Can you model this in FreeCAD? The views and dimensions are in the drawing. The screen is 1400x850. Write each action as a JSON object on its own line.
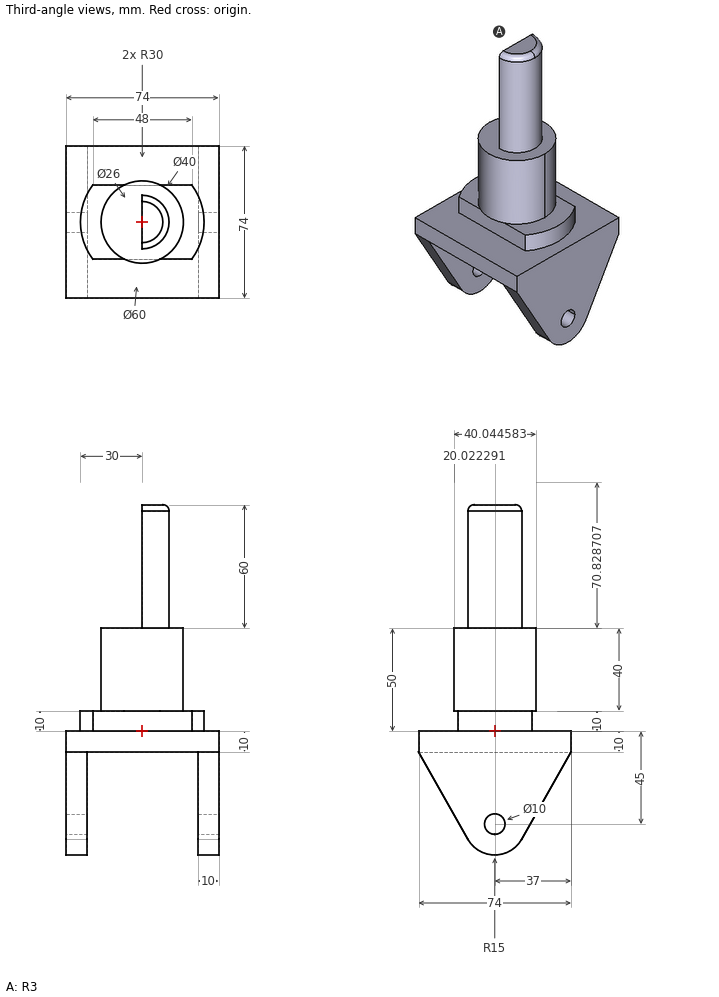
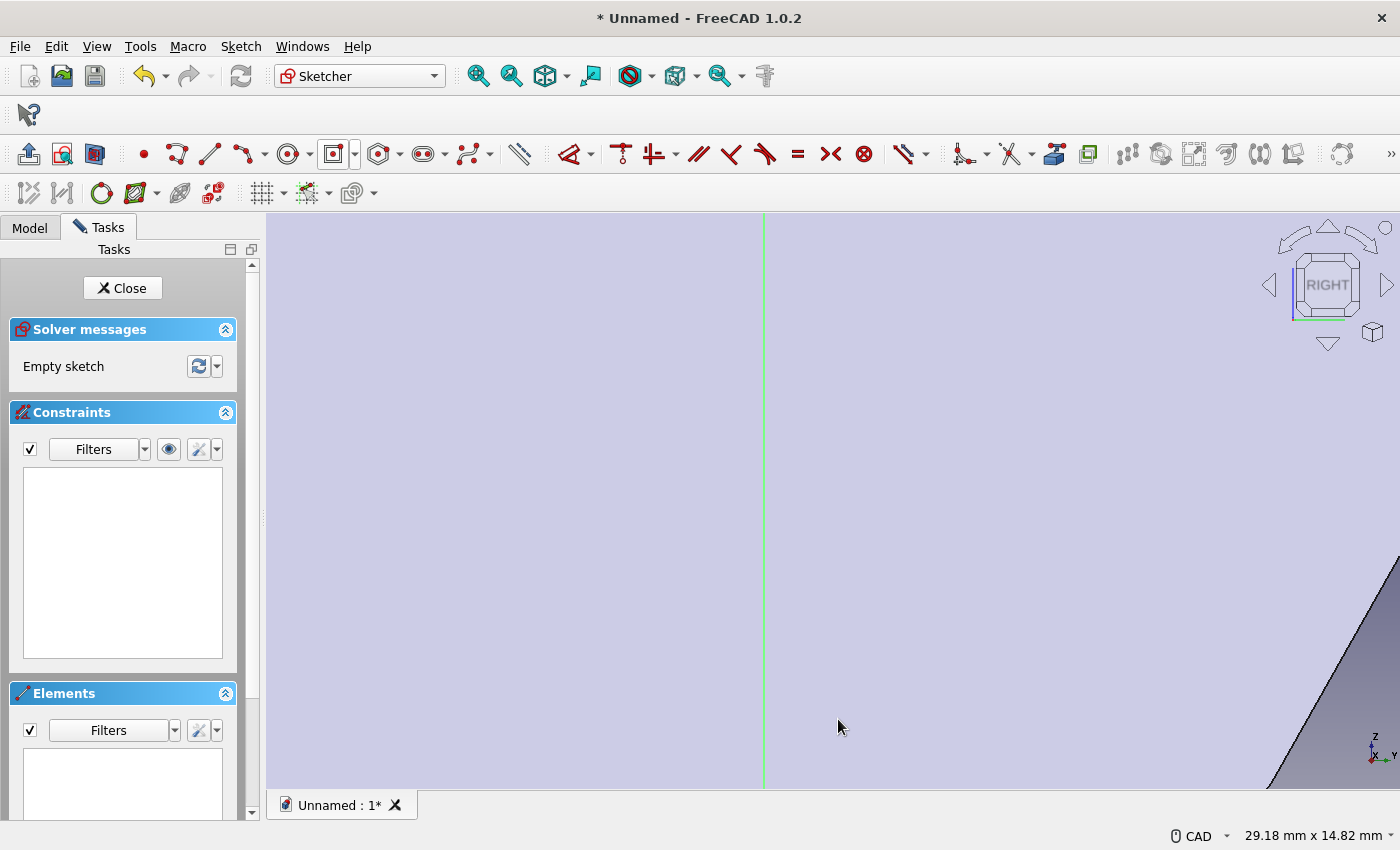
{"action": "left_click", "coordinate": [288, 154]}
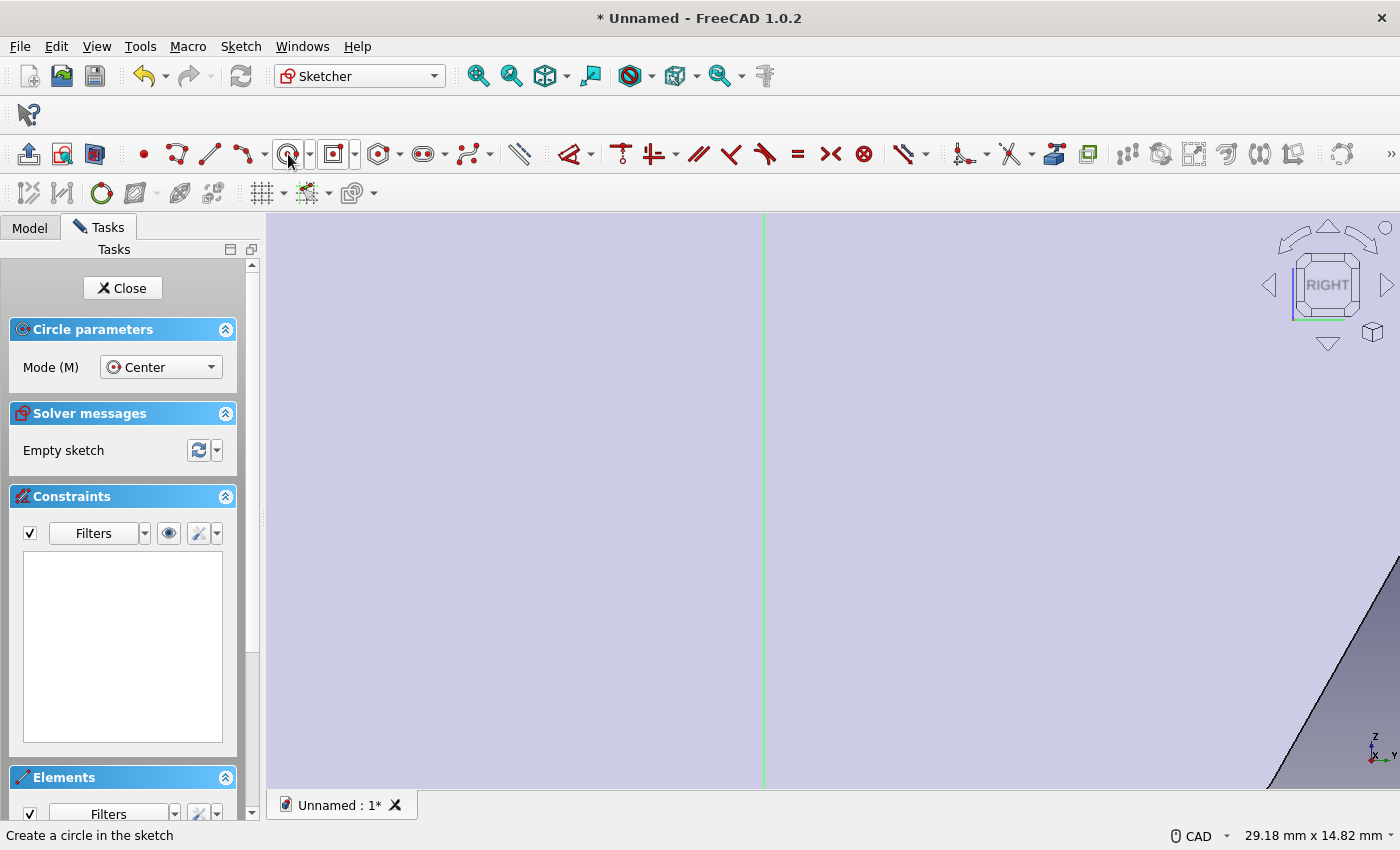
{"action": "left_click", "coordinate": [764, 495]}
{"action": "mouse_move", "coordinate": [902, 358]}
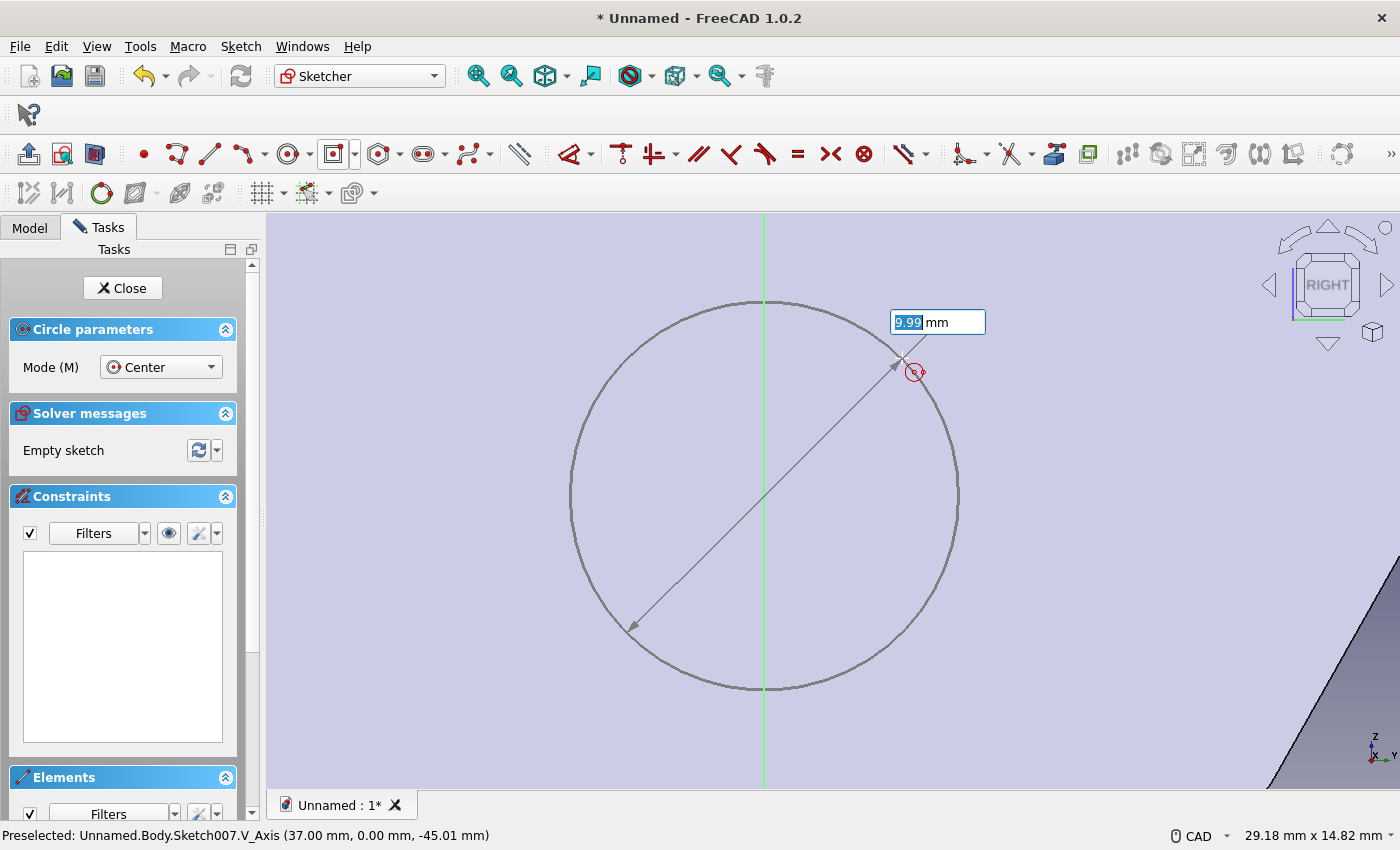
{"action": "type", "text": "10"}
{"action": "key", "text": "Return"}
{"action": "key", "text": "Escape"}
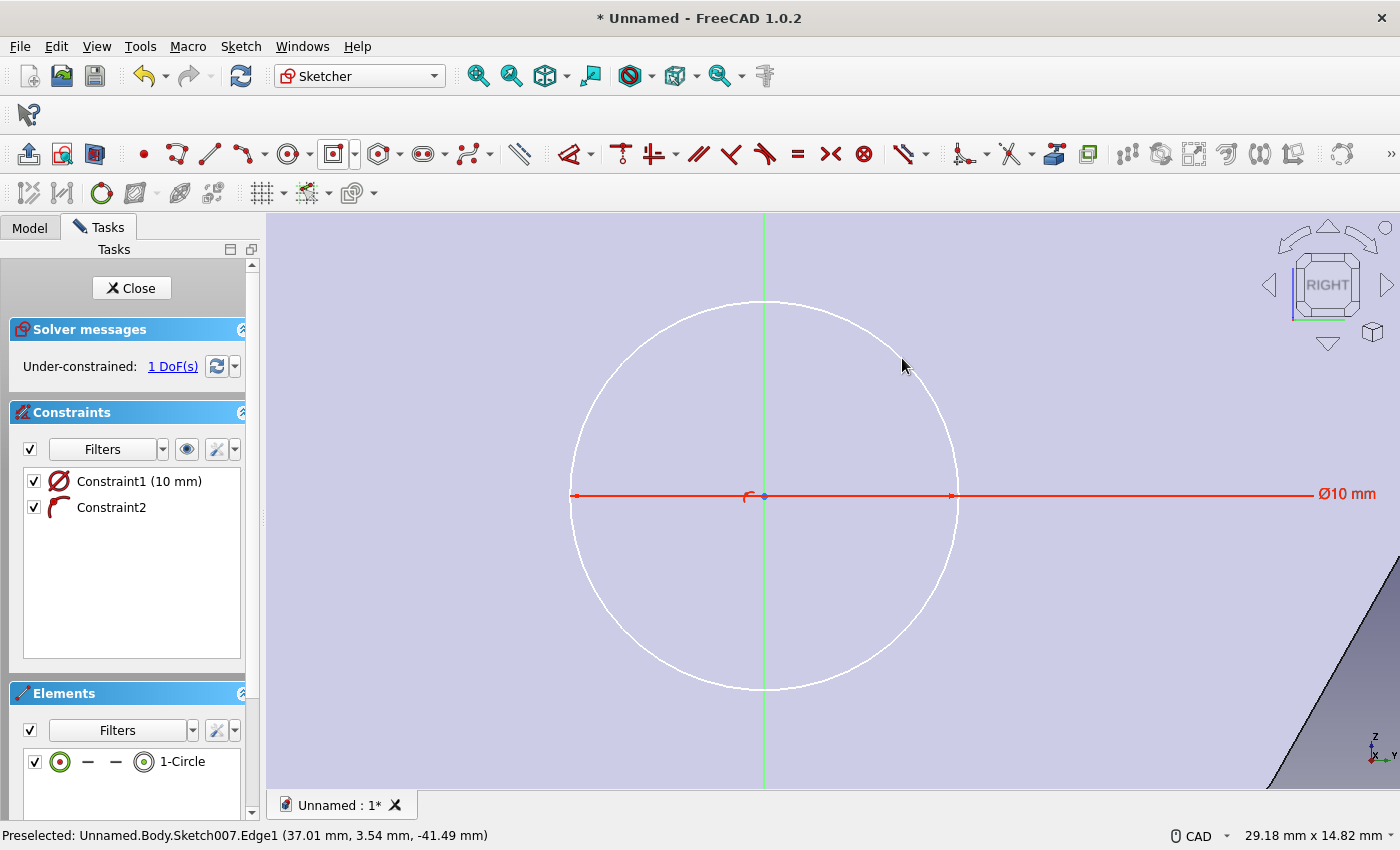
{"action": "key", "text": "d"}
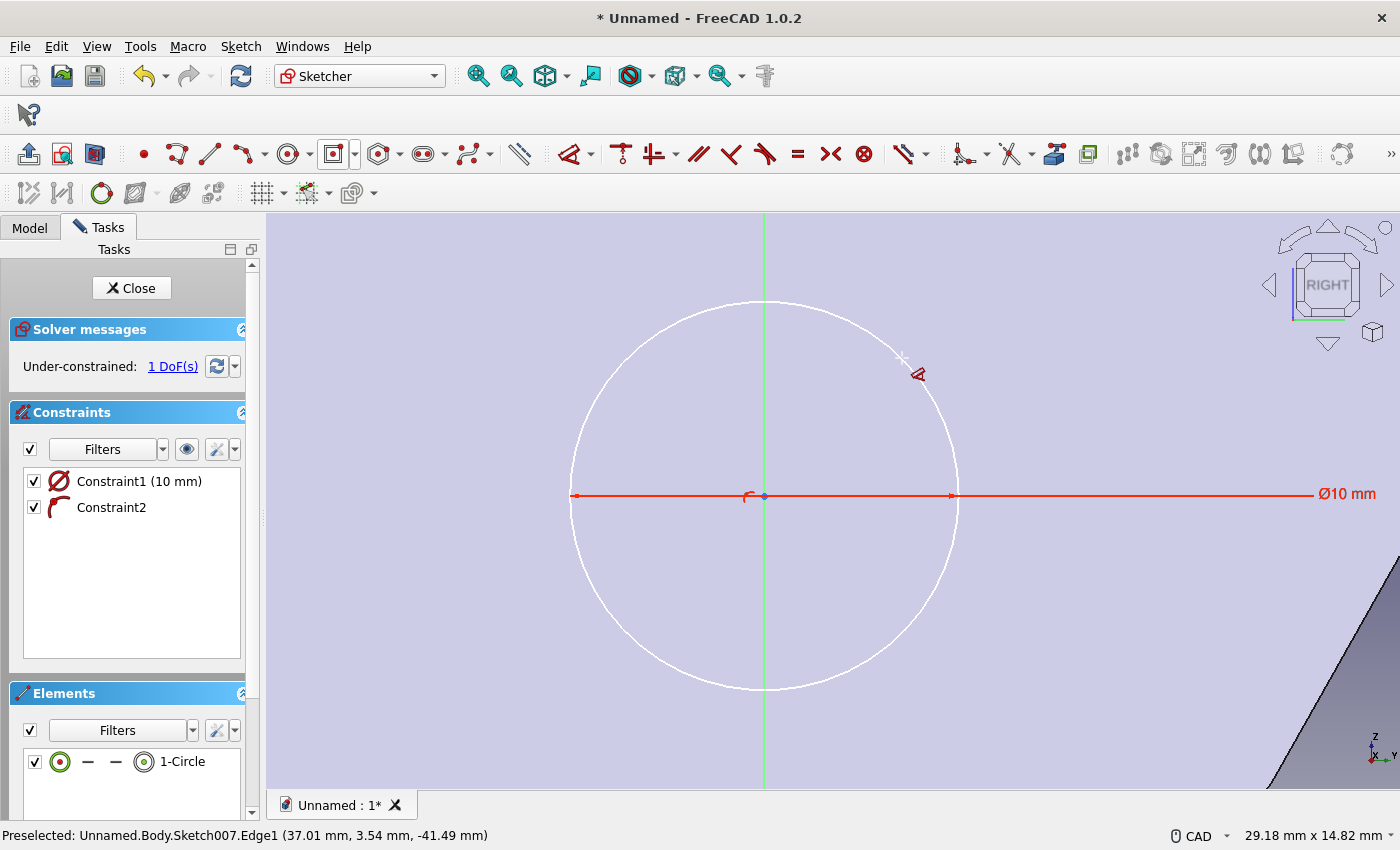
{"action": "left_click", "coordinate": [764, 496]}
{"action": "left_click", "coordinate": [798, 369]}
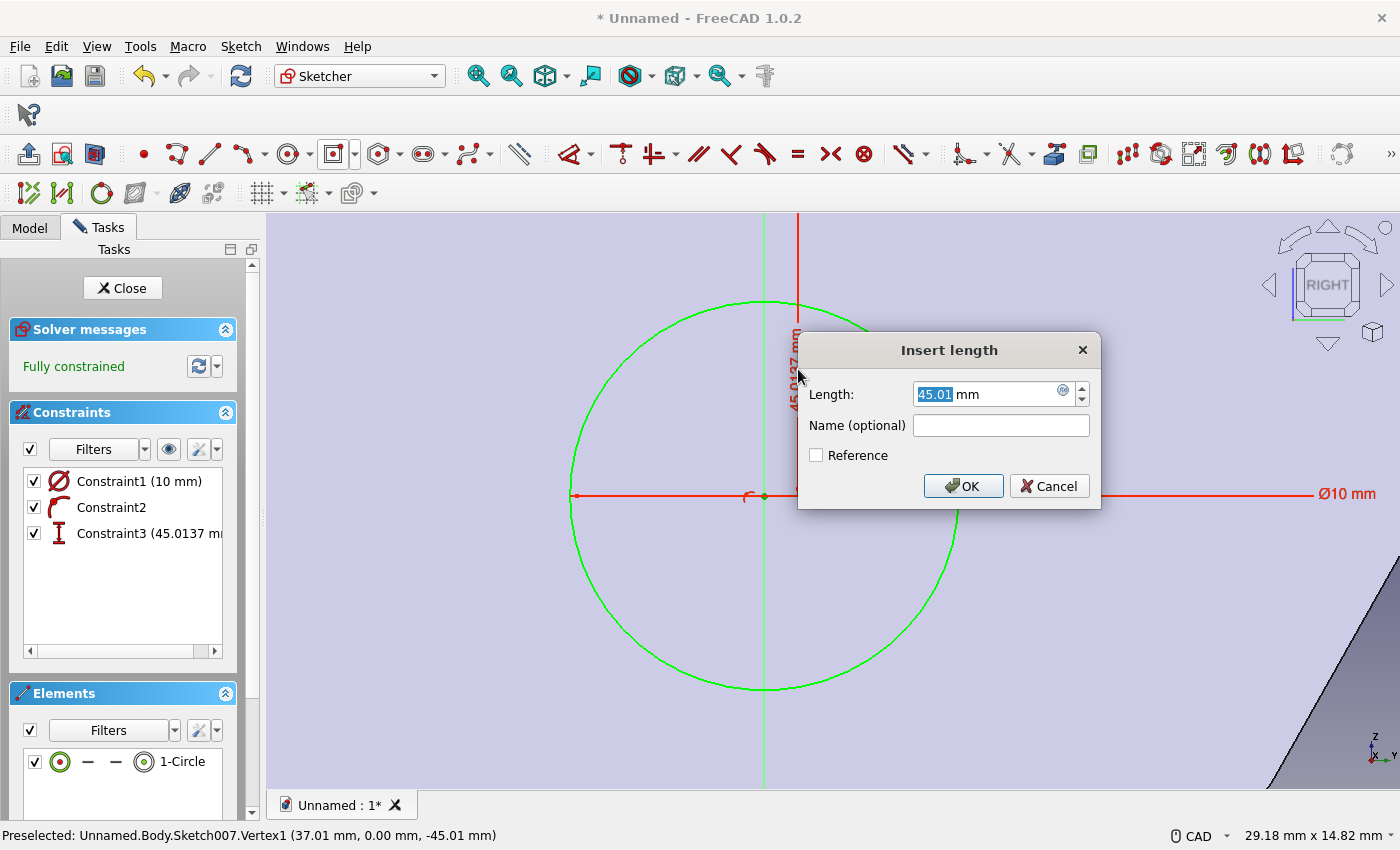
{"action": "type", "text": "45"}
{"action": "key", "text": "Return"}
{"action": "key", "text": "Escape"}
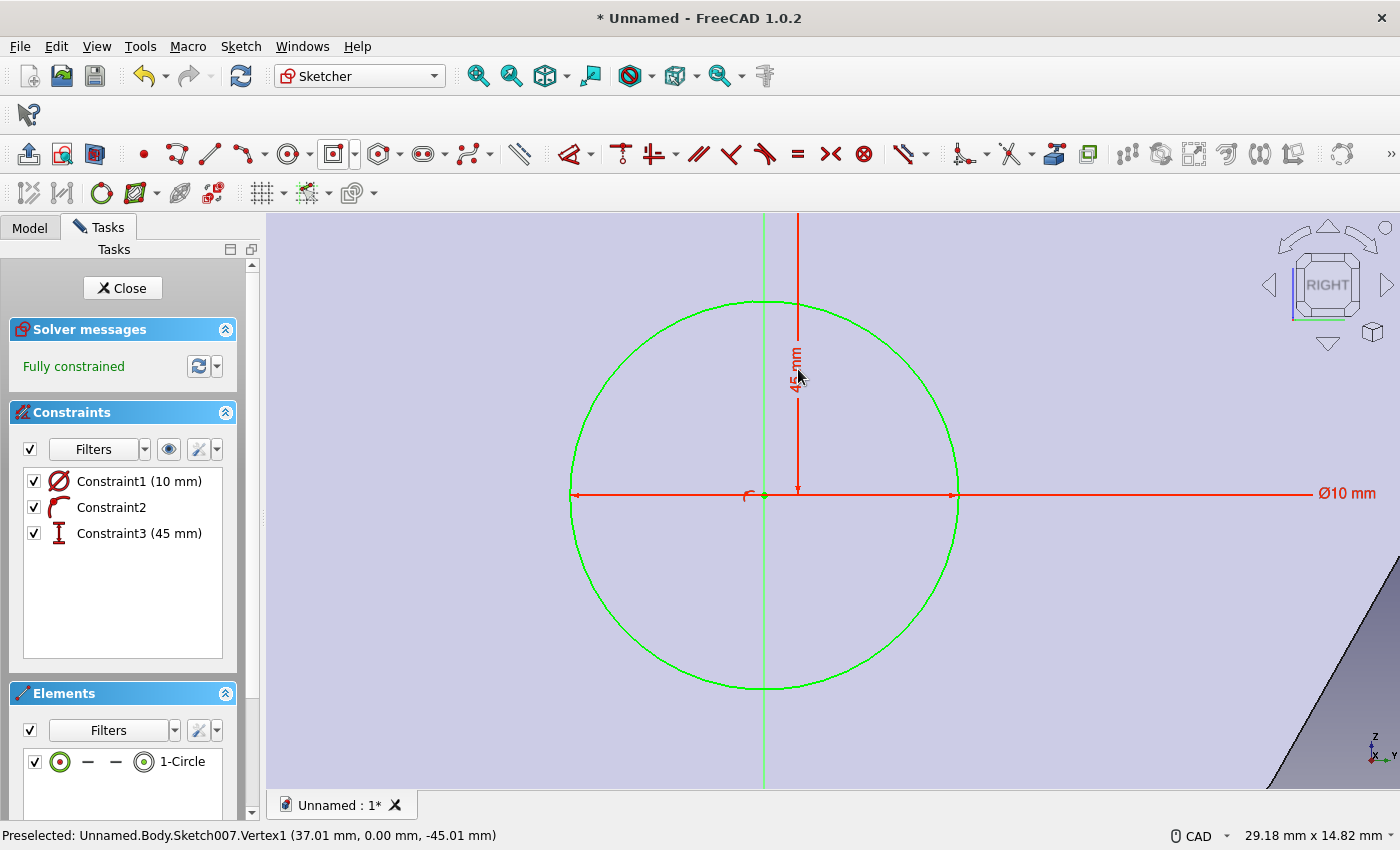
{"action": "left_click", "coordinate": [123, 288]}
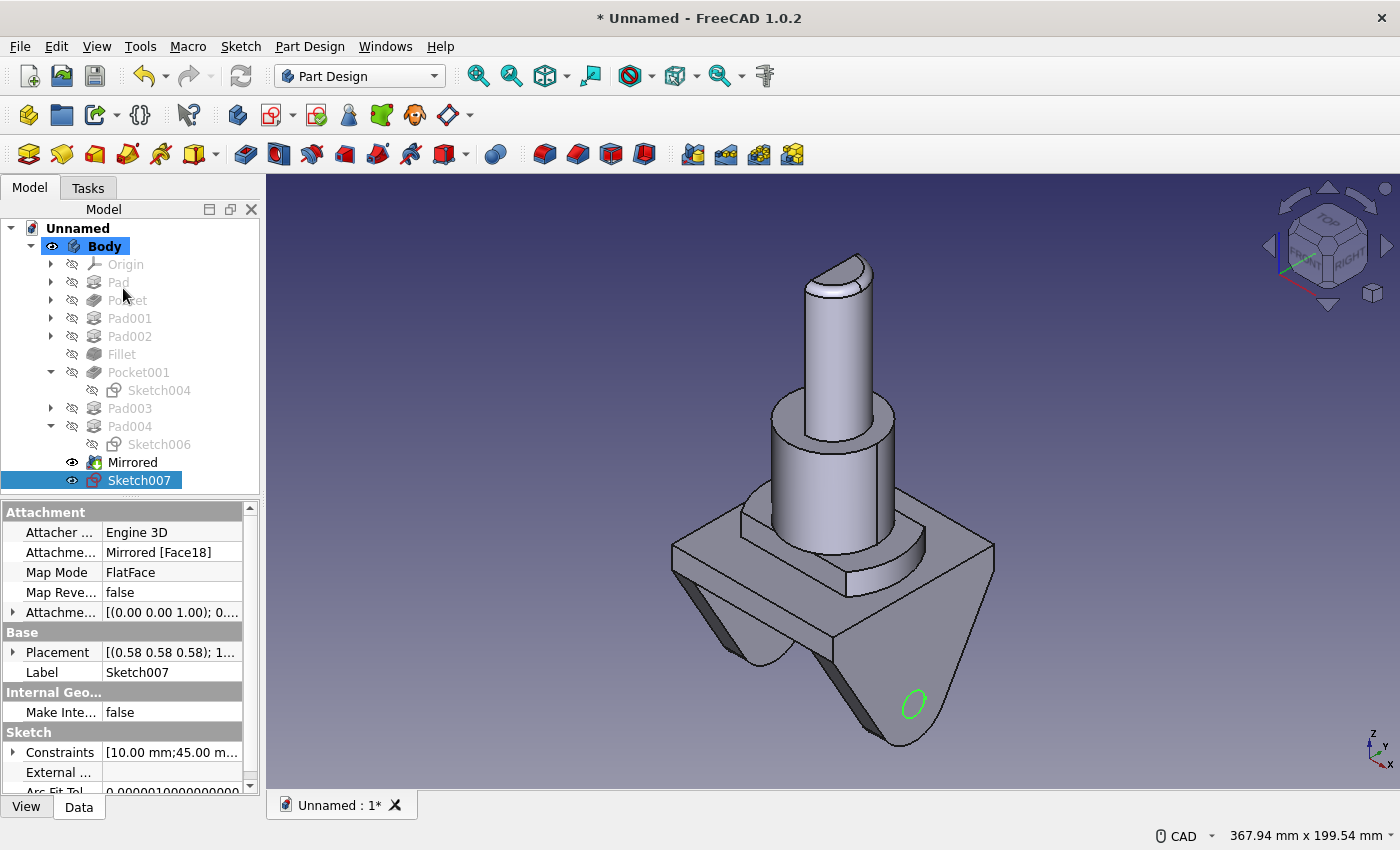
{"action": "left_click", "coordinate": [246, 154]}